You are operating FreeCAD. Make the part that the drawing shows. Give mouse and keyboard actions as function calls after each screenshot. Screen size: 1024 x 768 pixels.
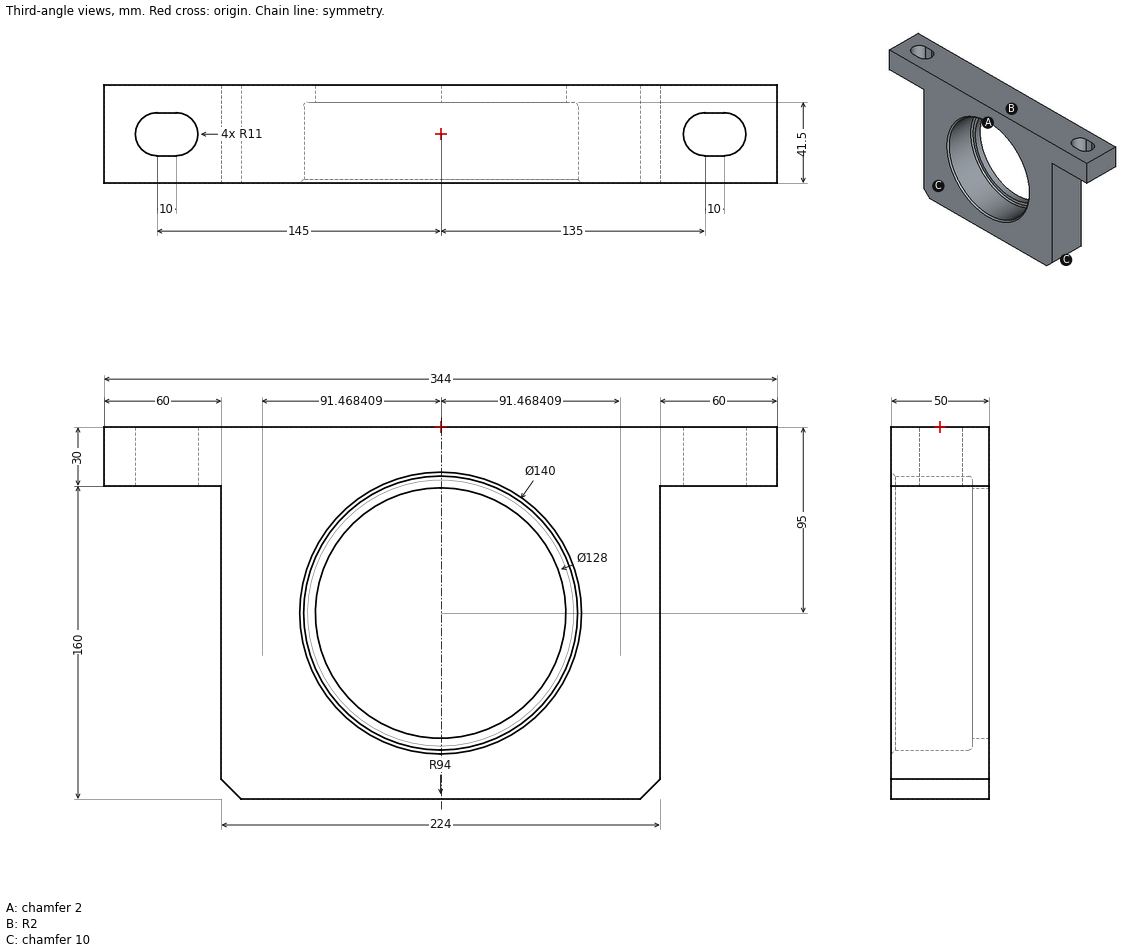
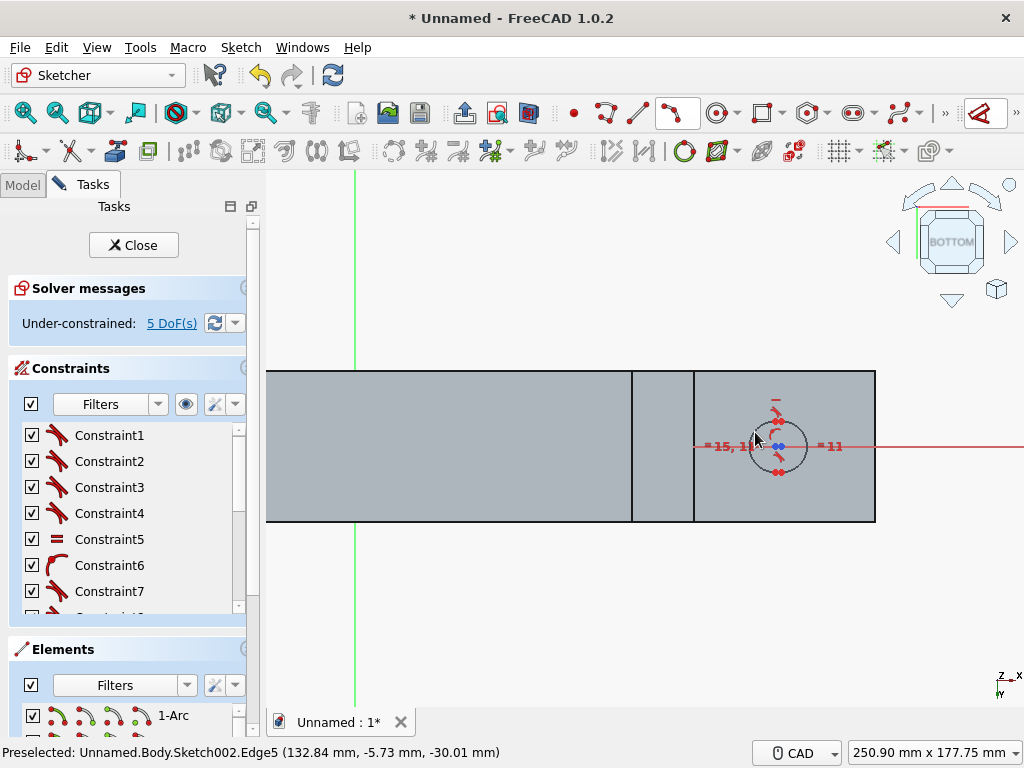
key(d)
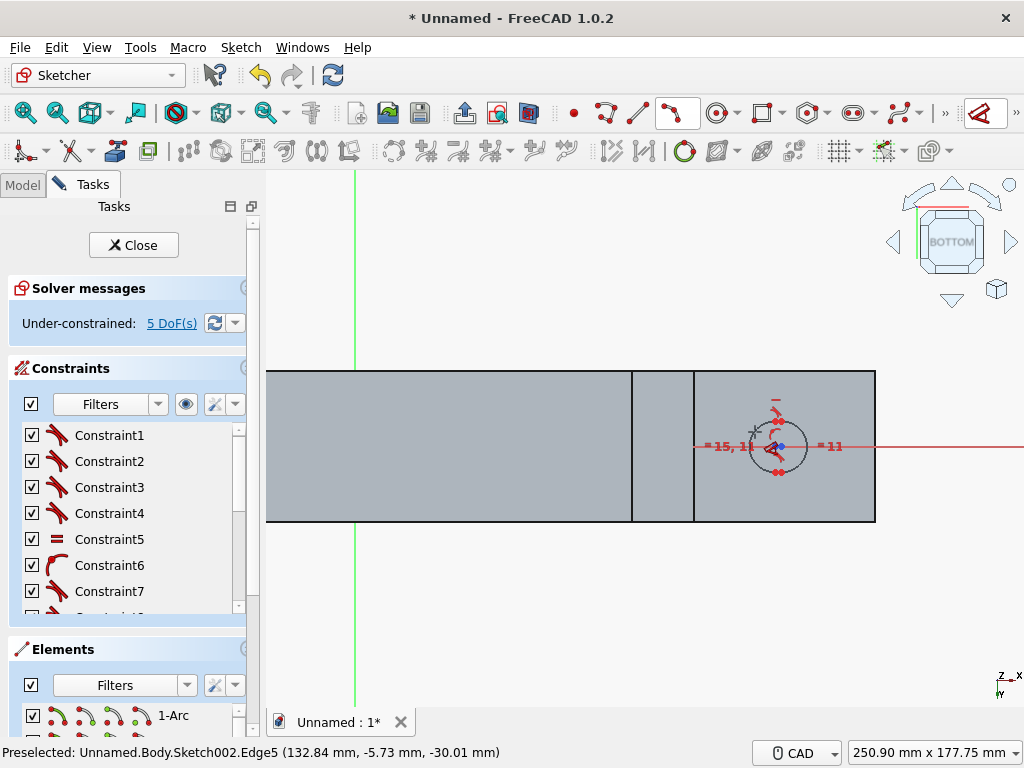
scroll(757, 432, down, 4)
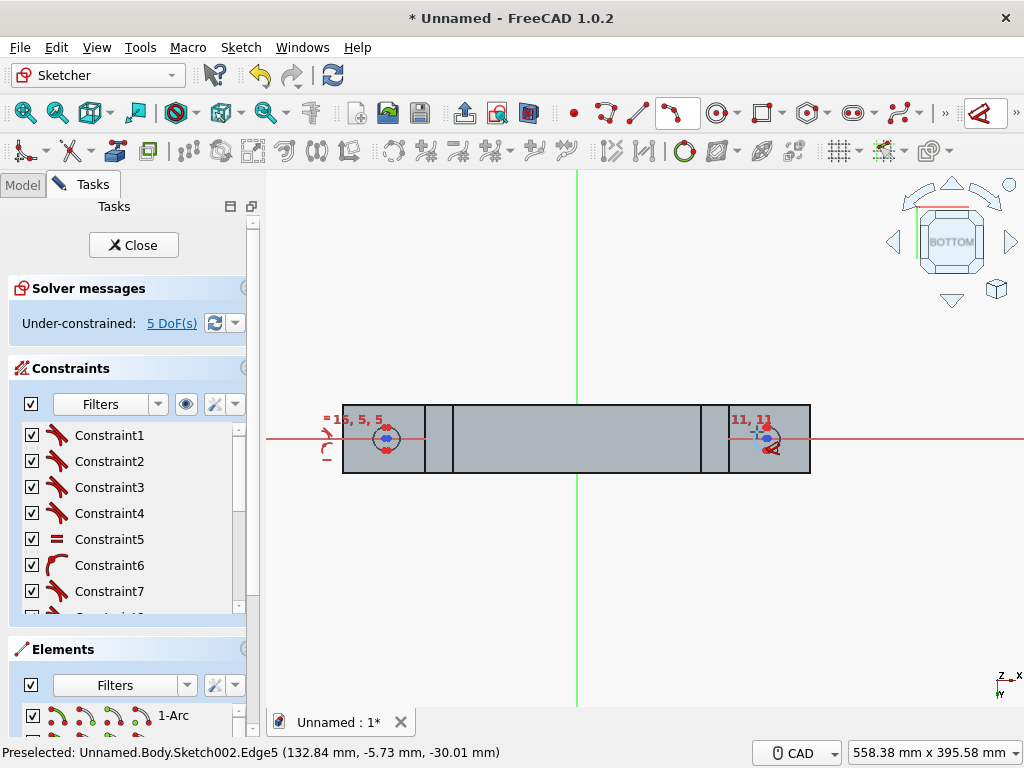
scroll(376, 432, up, 5)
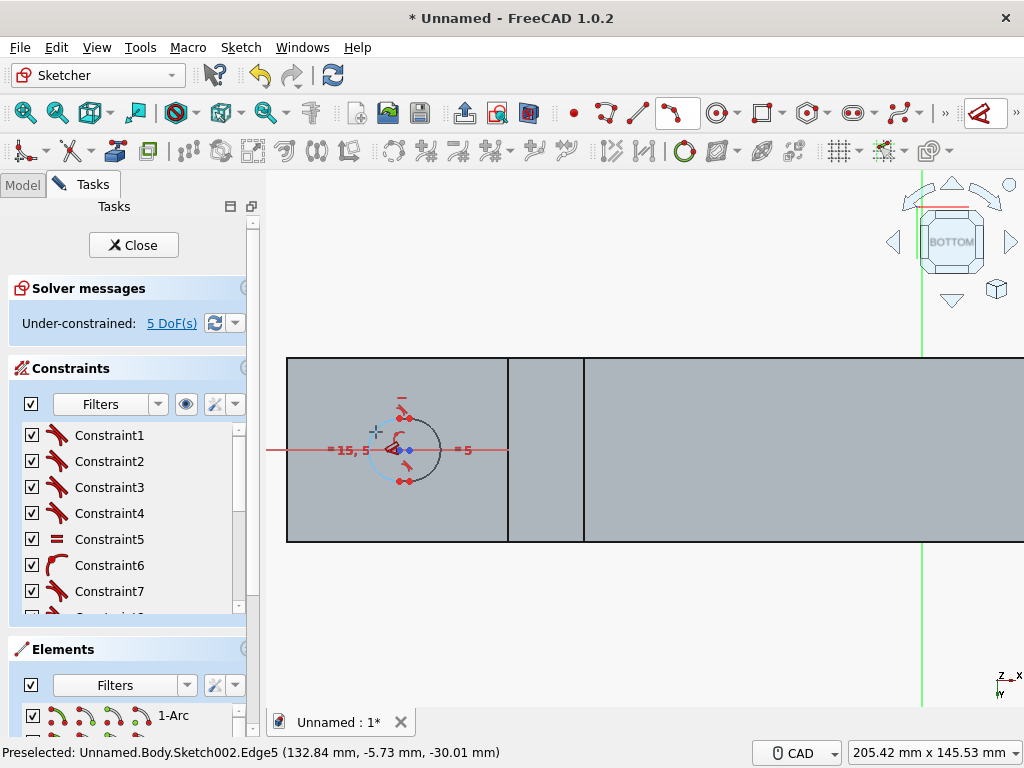
click(375, 432)
click(349, 413)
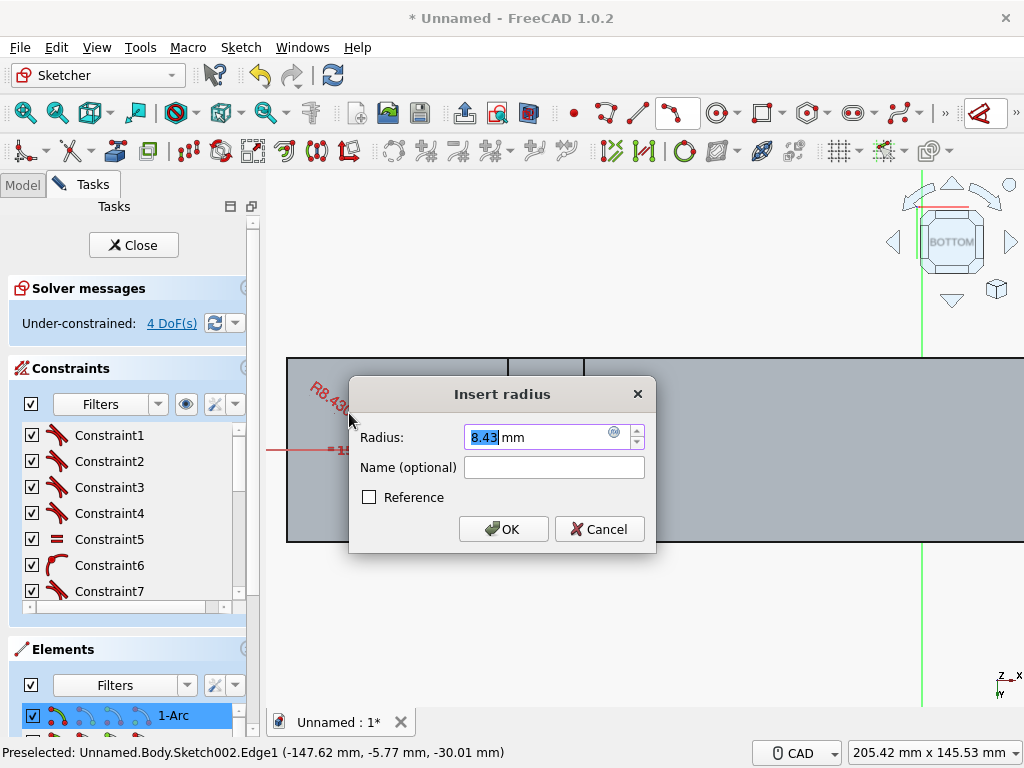
text(11)
key(Return)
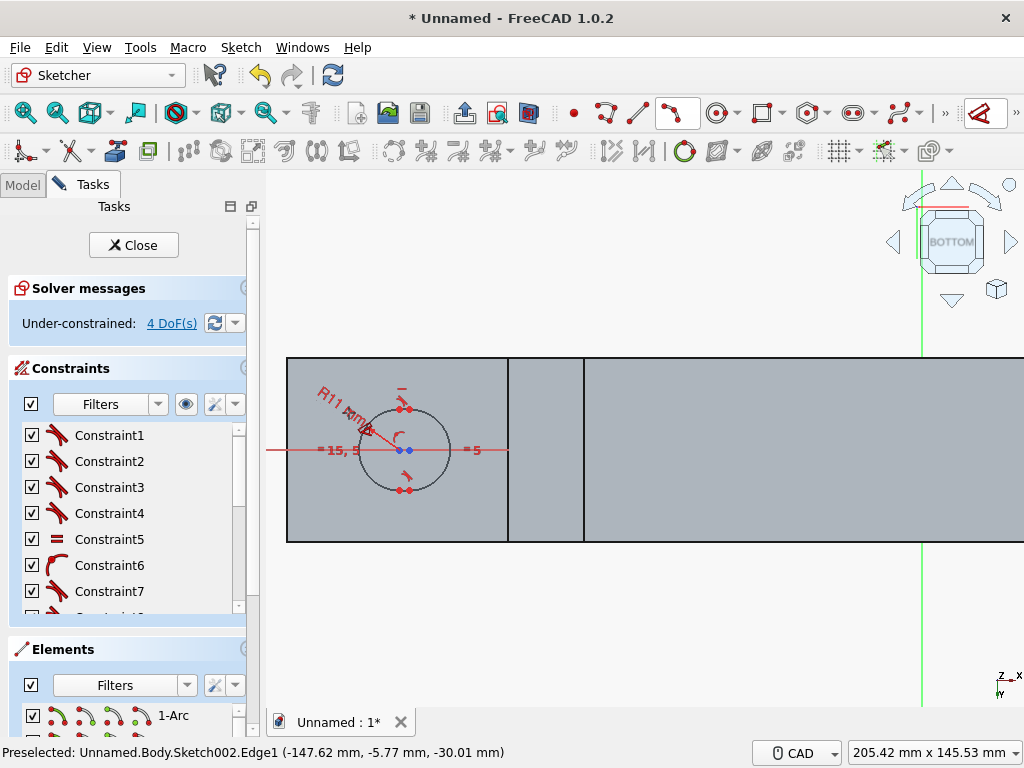
scroll(405, 409, up, 6)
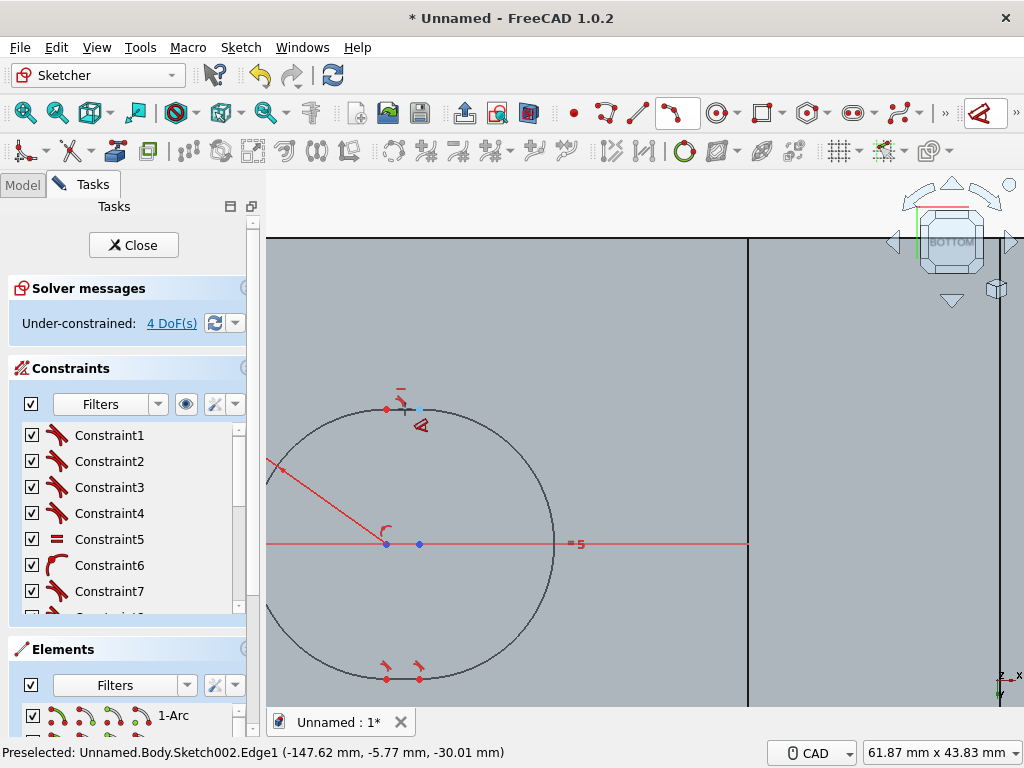
click(403, 410)
click(403, 376)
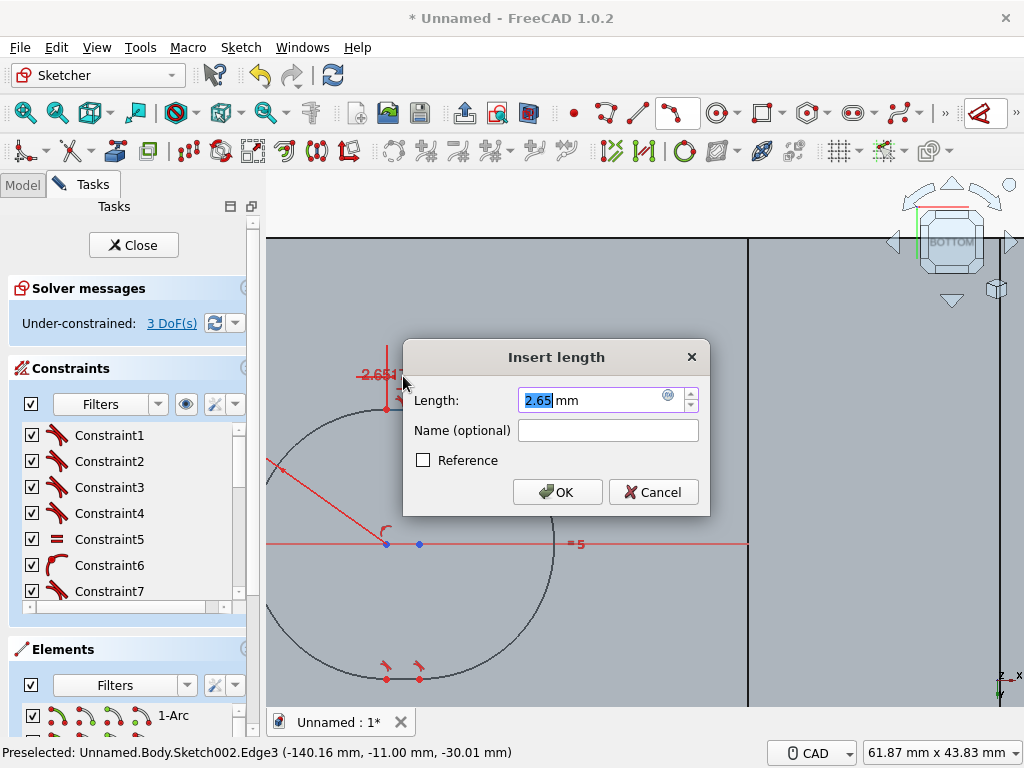
text(10)
key(Return)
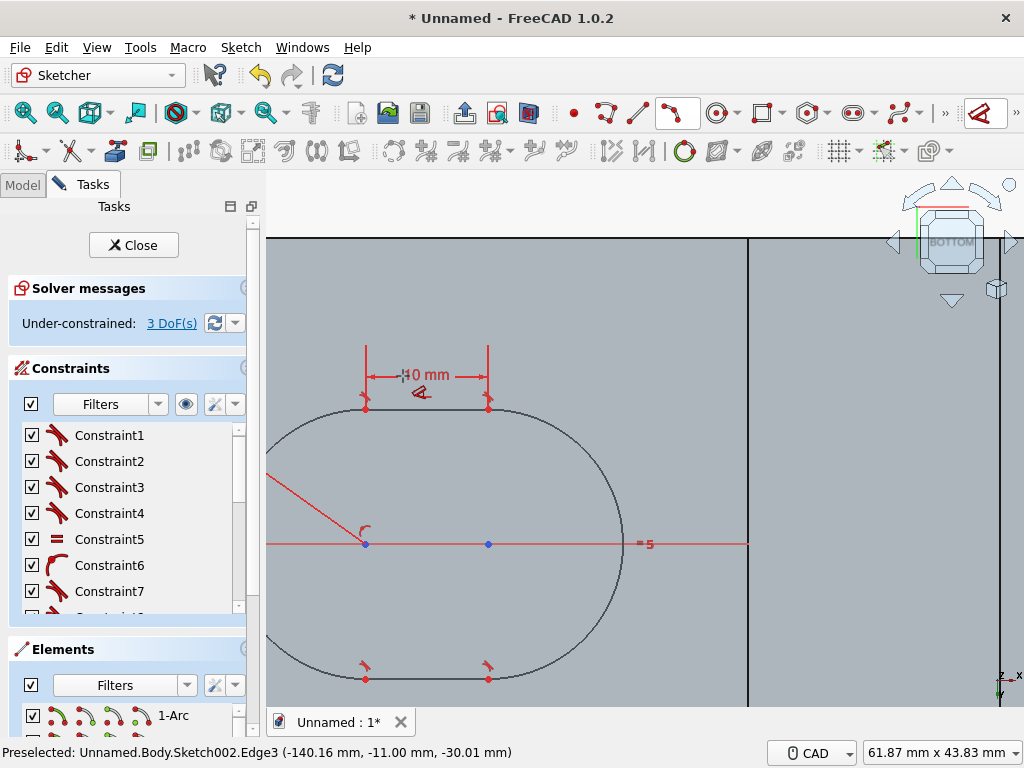
scroll(384, 425, down, 11)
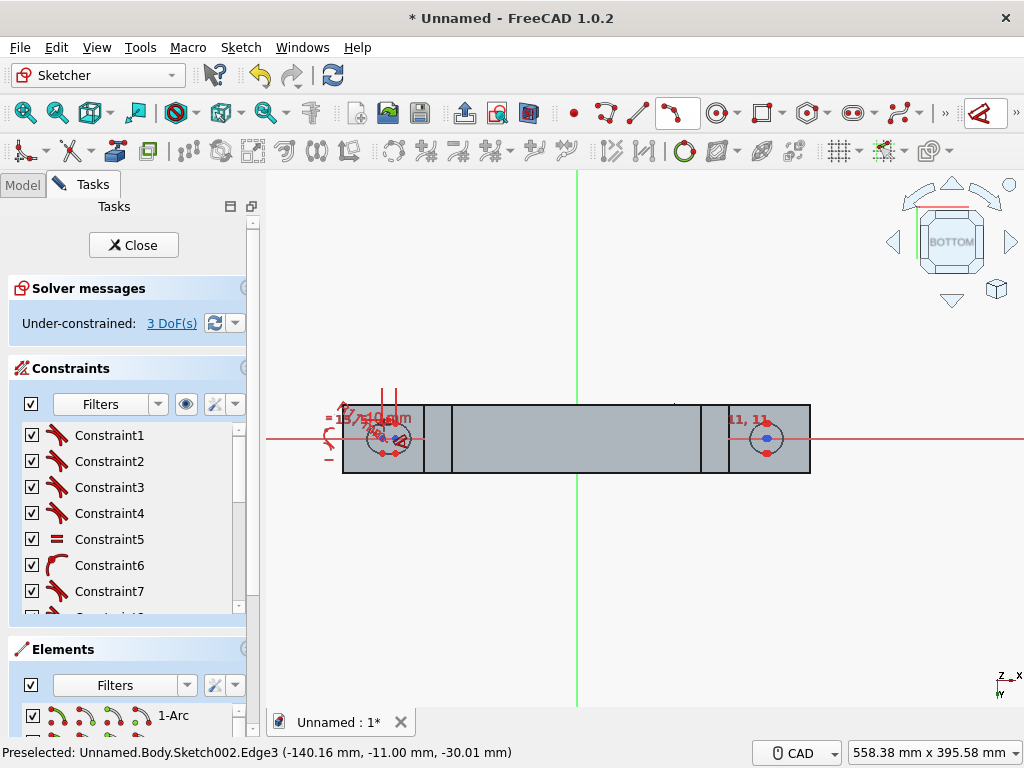
scroll(766, 424, up, 13)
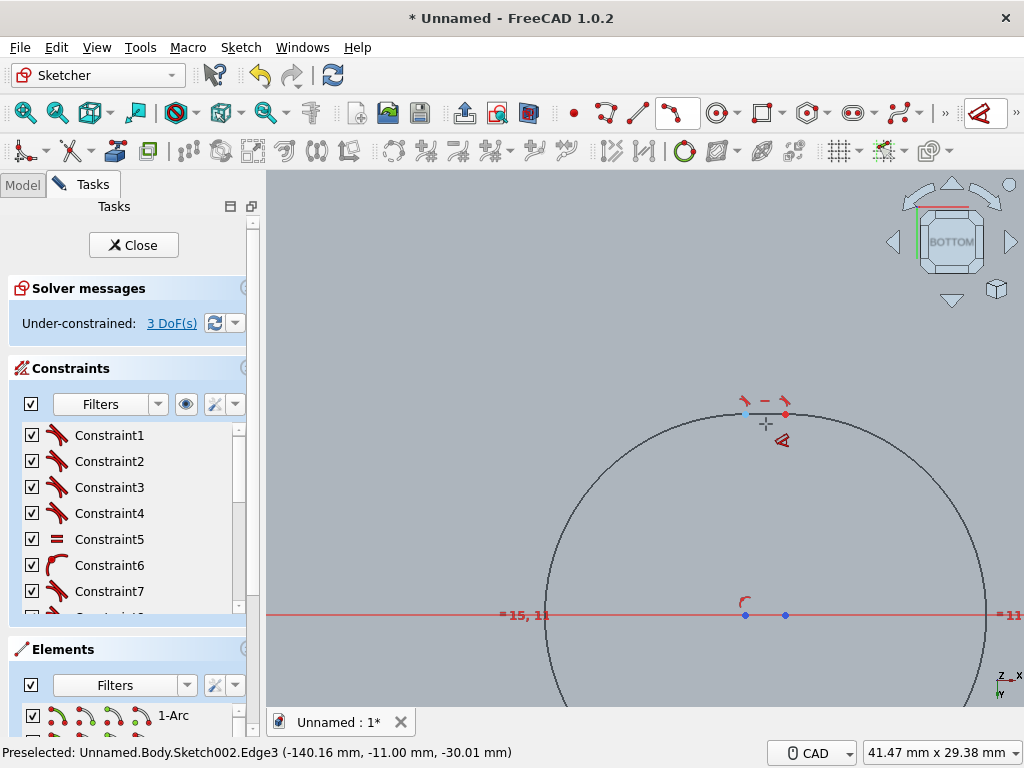
click(762, 414)
click(766, 380)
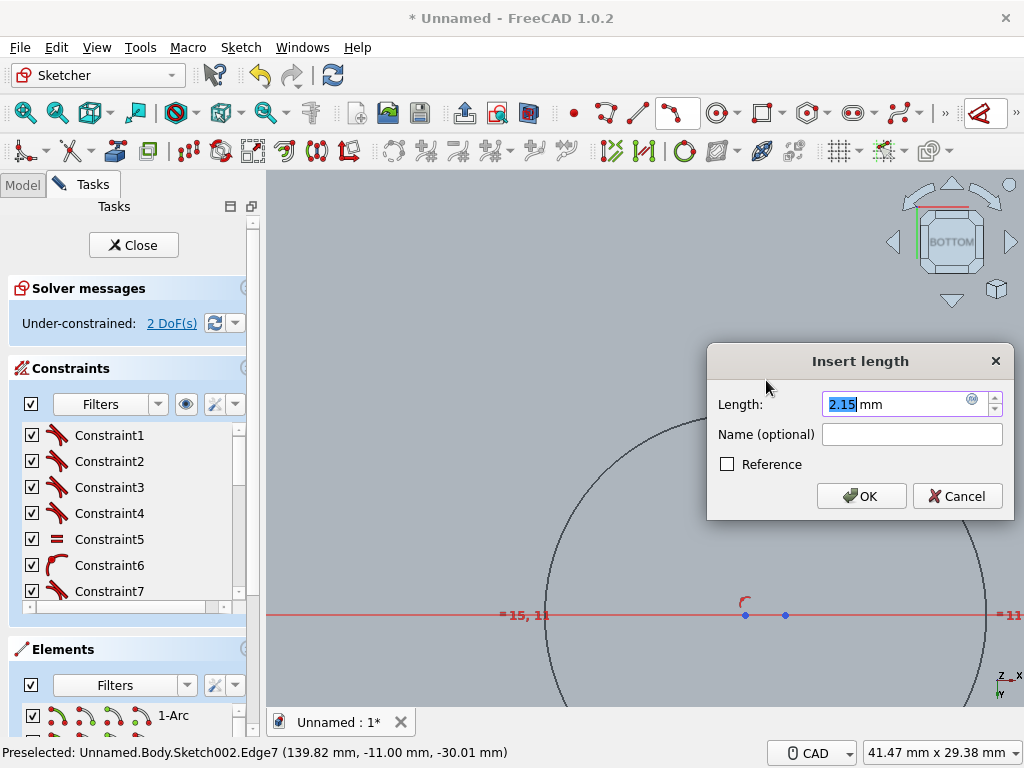
text(10)
key(Return)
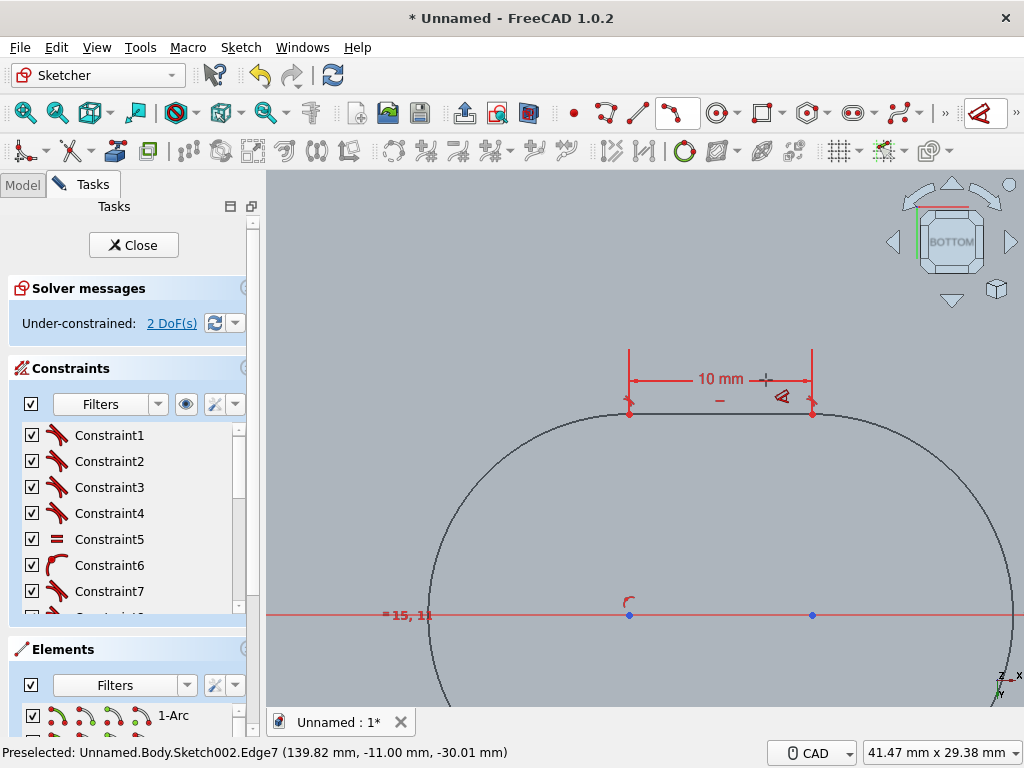
scroll(767, 424, down, 13)